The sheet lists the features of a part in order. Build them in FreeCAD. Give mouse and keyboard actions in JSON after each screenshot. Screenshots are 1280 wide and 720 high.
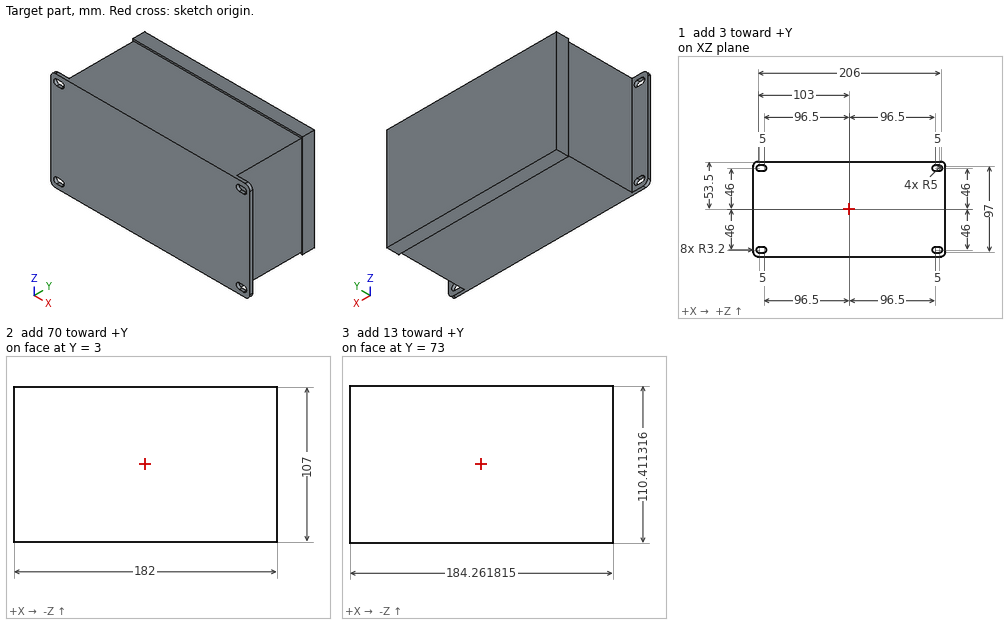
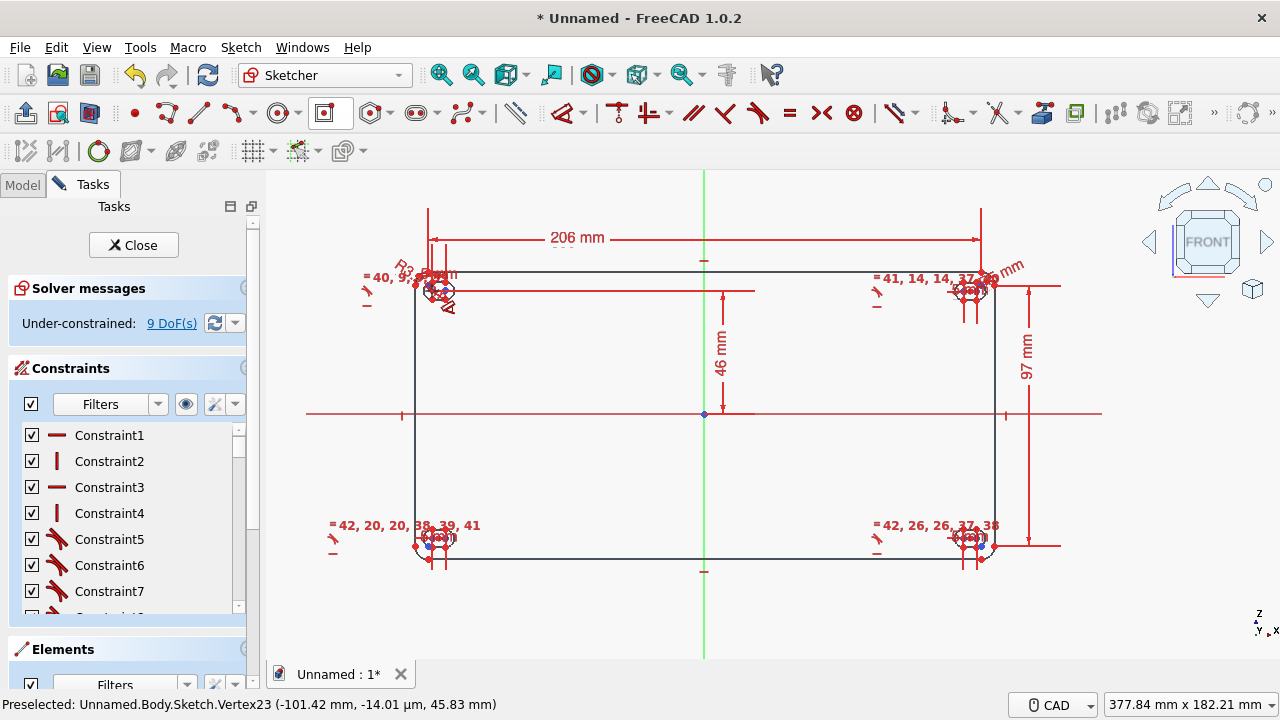
{"action": "scroll", "coordinate": [964, 292], "scroll_direction": "up", "scroll_amount": 2}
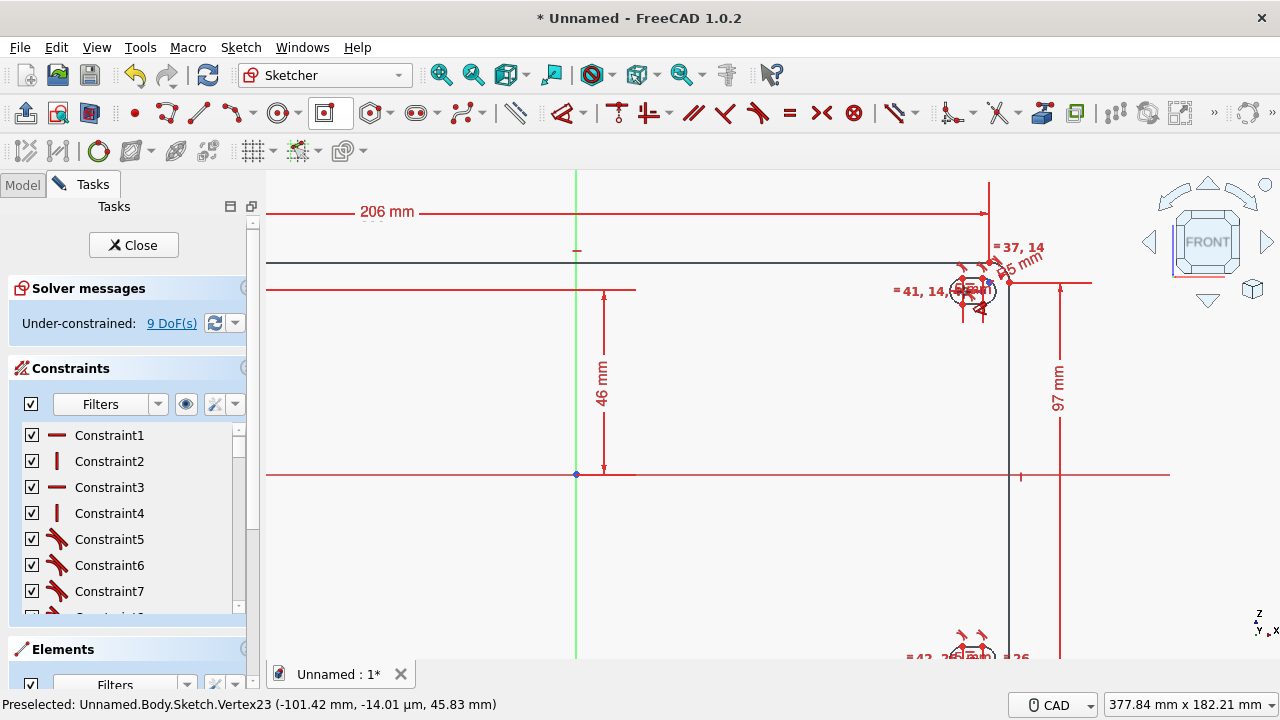
{"action": "left_click", "coordinate": [963, 291]}
{"action": "left_click", "coordinate": [542, 341]}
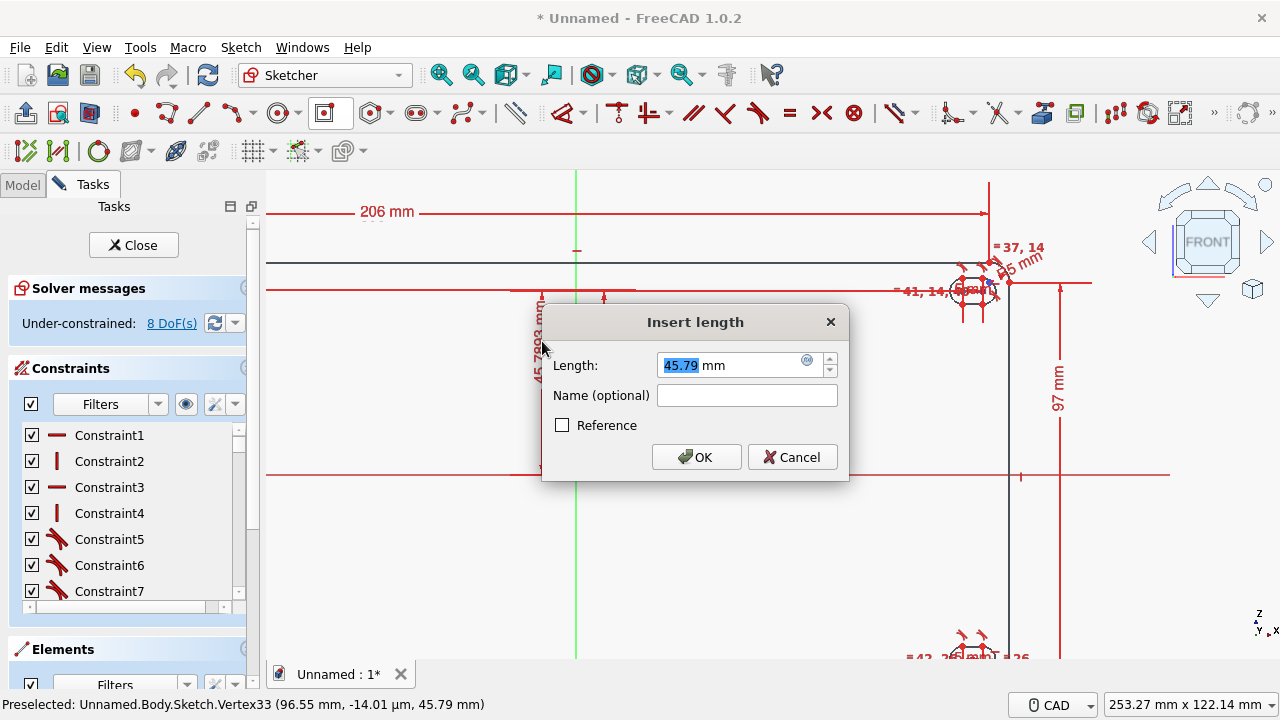
{"action": "type", "text": "46"}
{"action": "key", "text": "Return"}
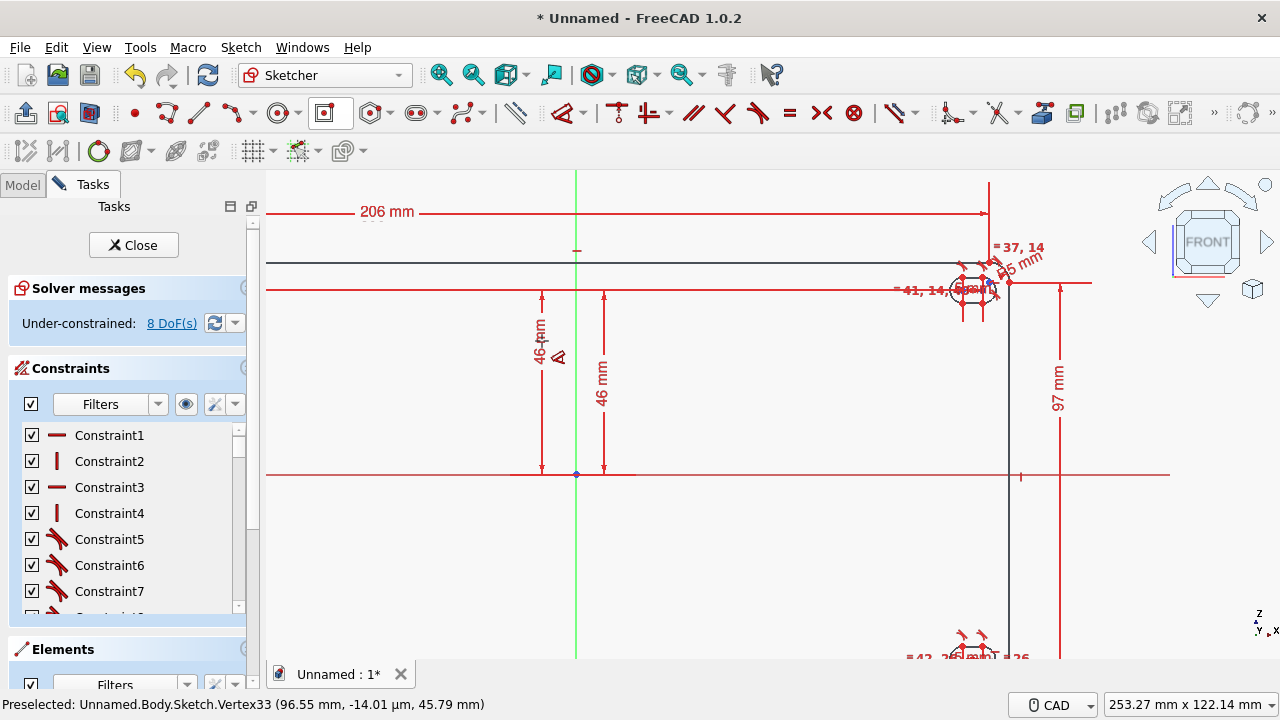
{"action": "scroll", "coordinate": [965, 292], "scroll_direction": "down", "scroll_amount": 2}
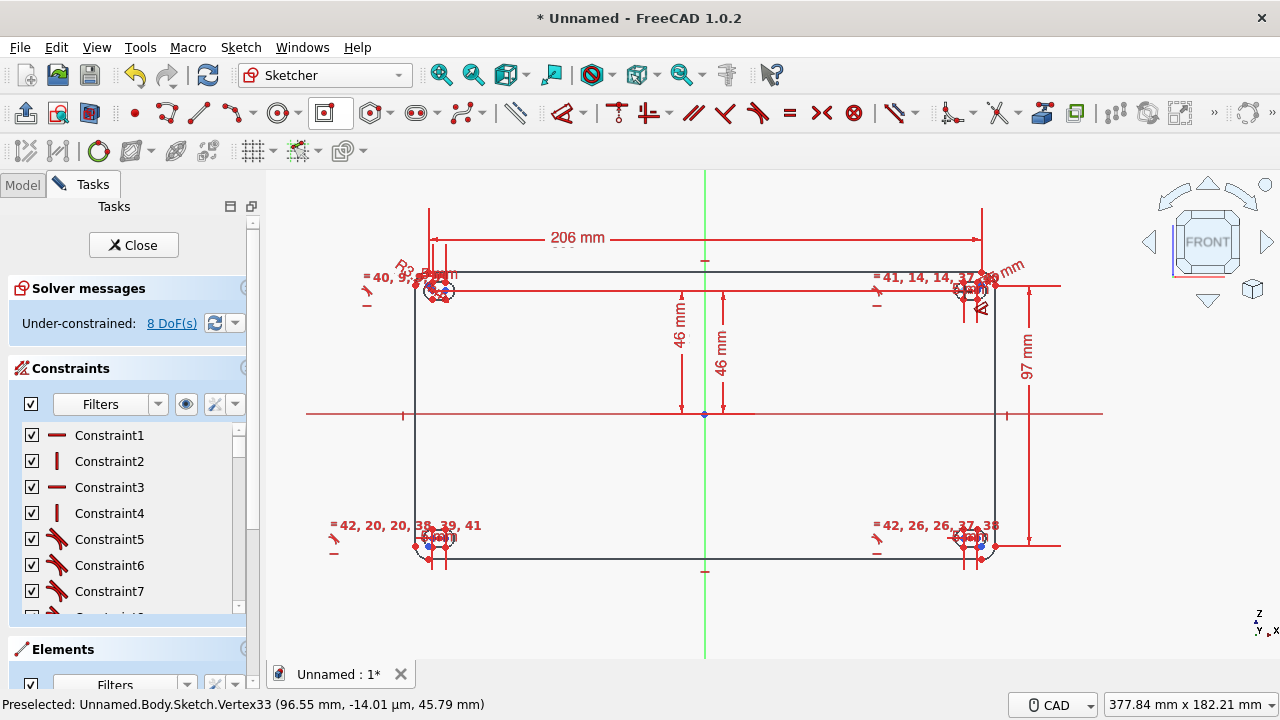
{"action": "scroll", "coordinate": [432, 539], "scroll_direction": "up", "scroll_amount": 2}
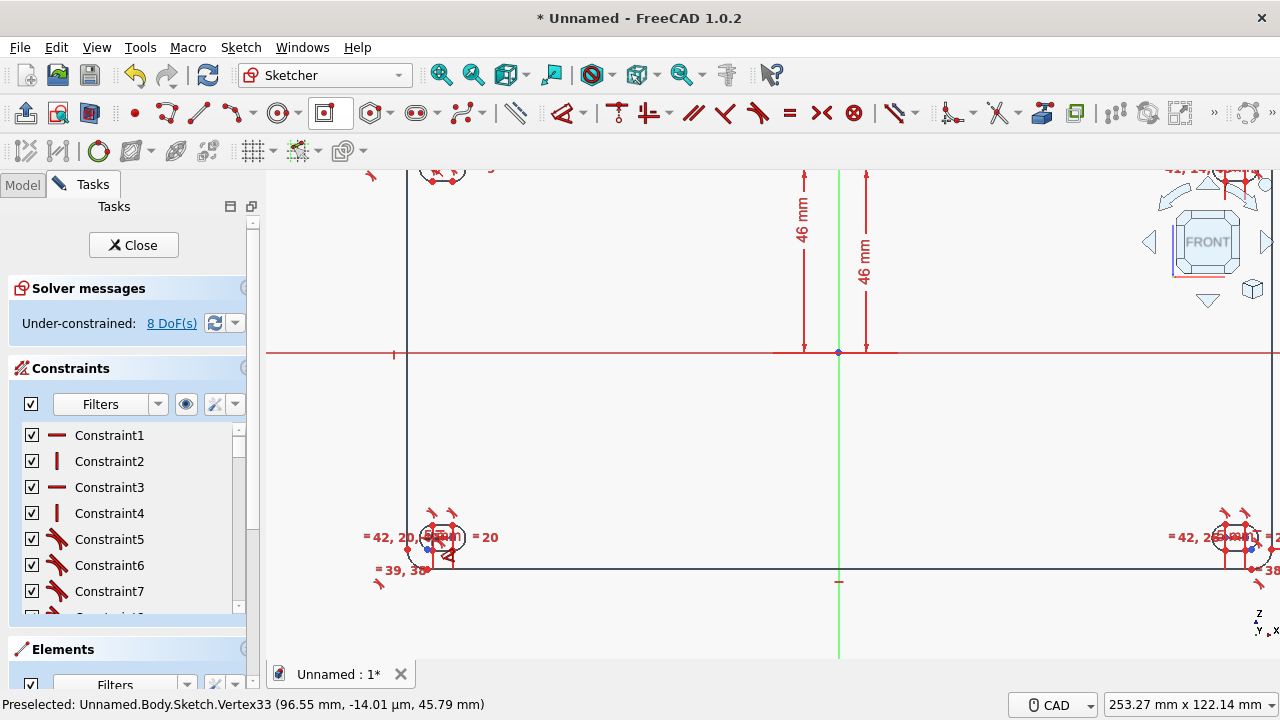
{"action": "left_click", "coordinate": [433, 538]}
{"action": "left_click", "coordinate": [873, 445]}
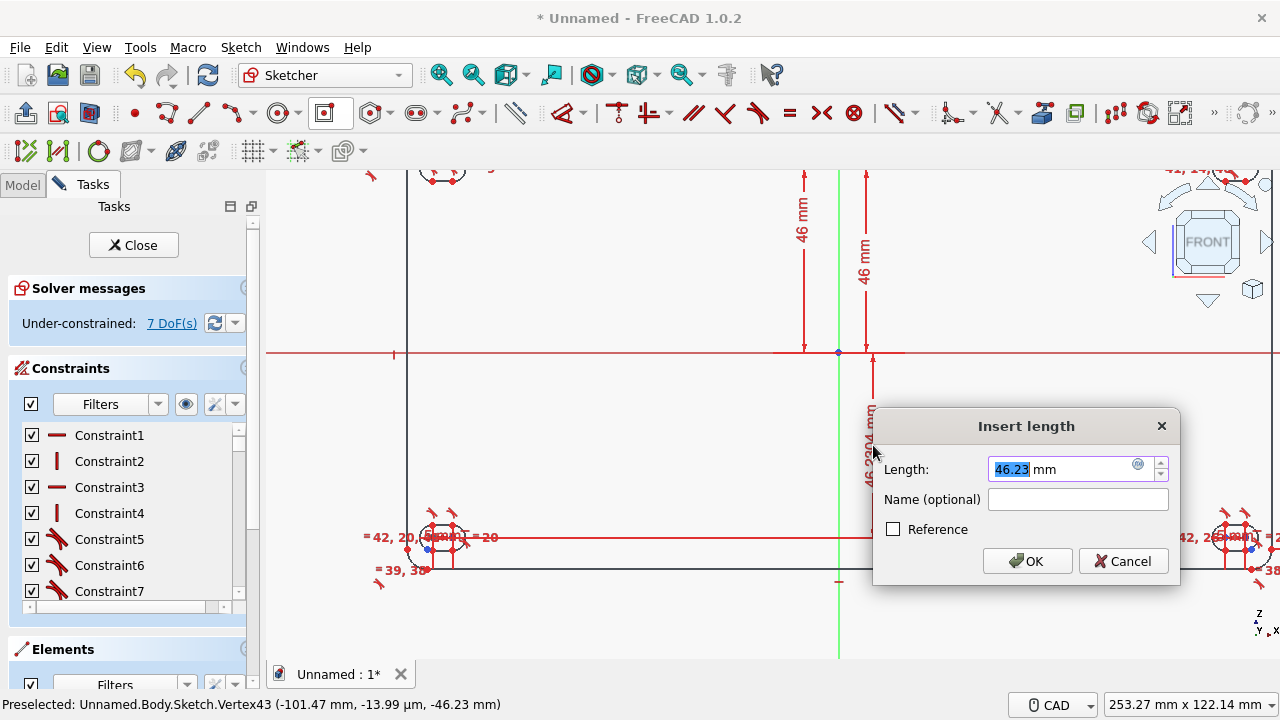
{"action": "type", "text": "46"}
{"action": "key", "text": "Return"}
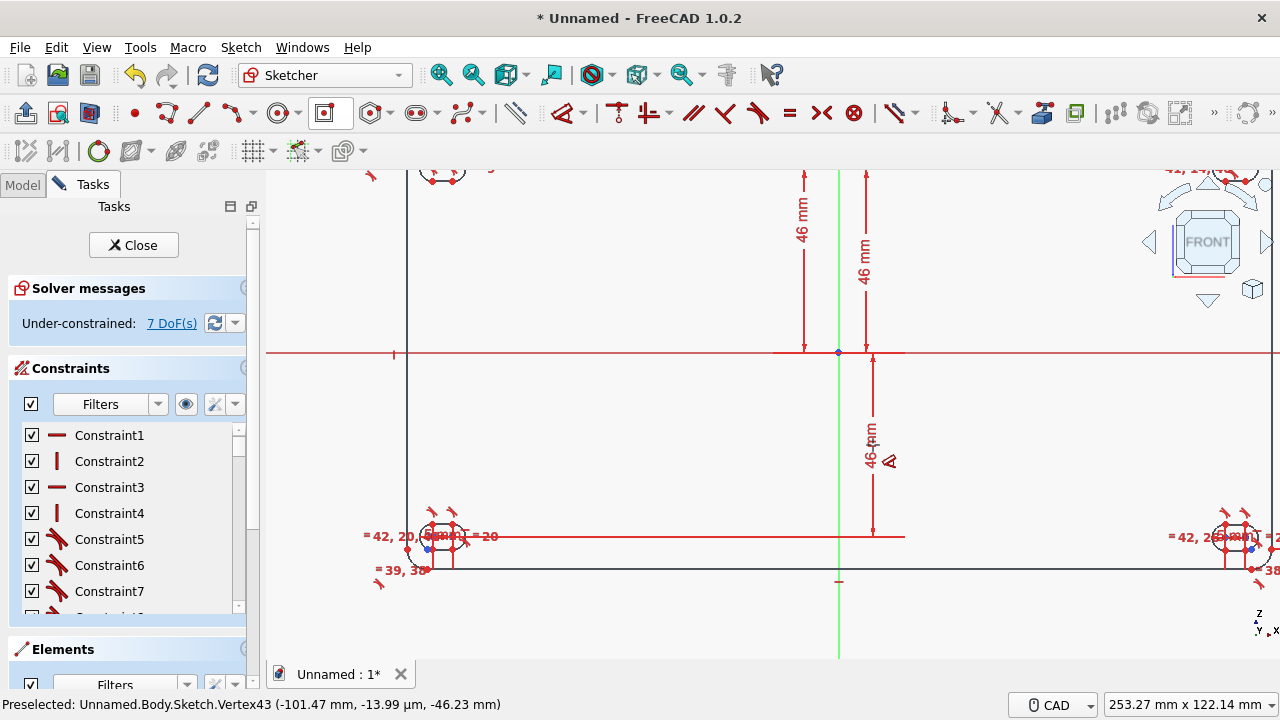
{"action": "scroll", "coordinate": [431, 540], "scroll_direction": "down", "scroll_amount": 2}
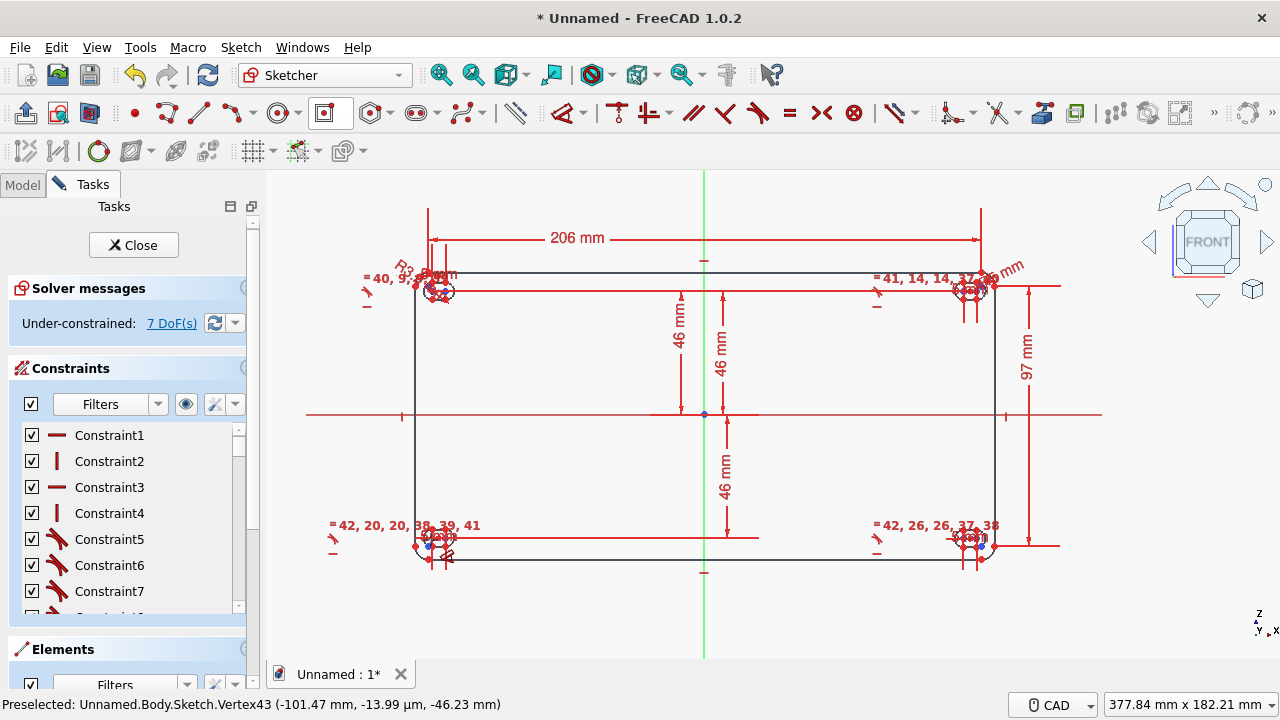
{"action": "scroll", "coordinate": [963, 539], "scroll_direction": "up", "scroll_amount": 2}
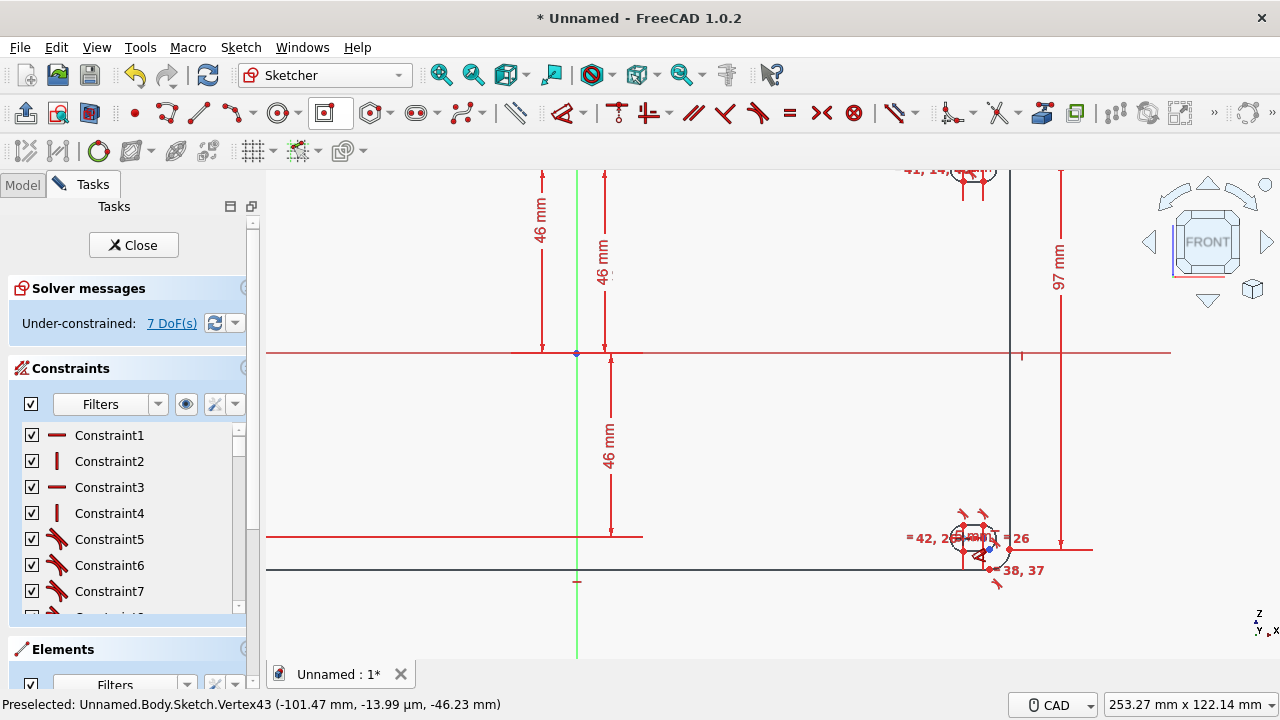
{"action": "left_click", "coordinate": [963, 538]}
{"action": "left_click", "coordinate": [543, 403]}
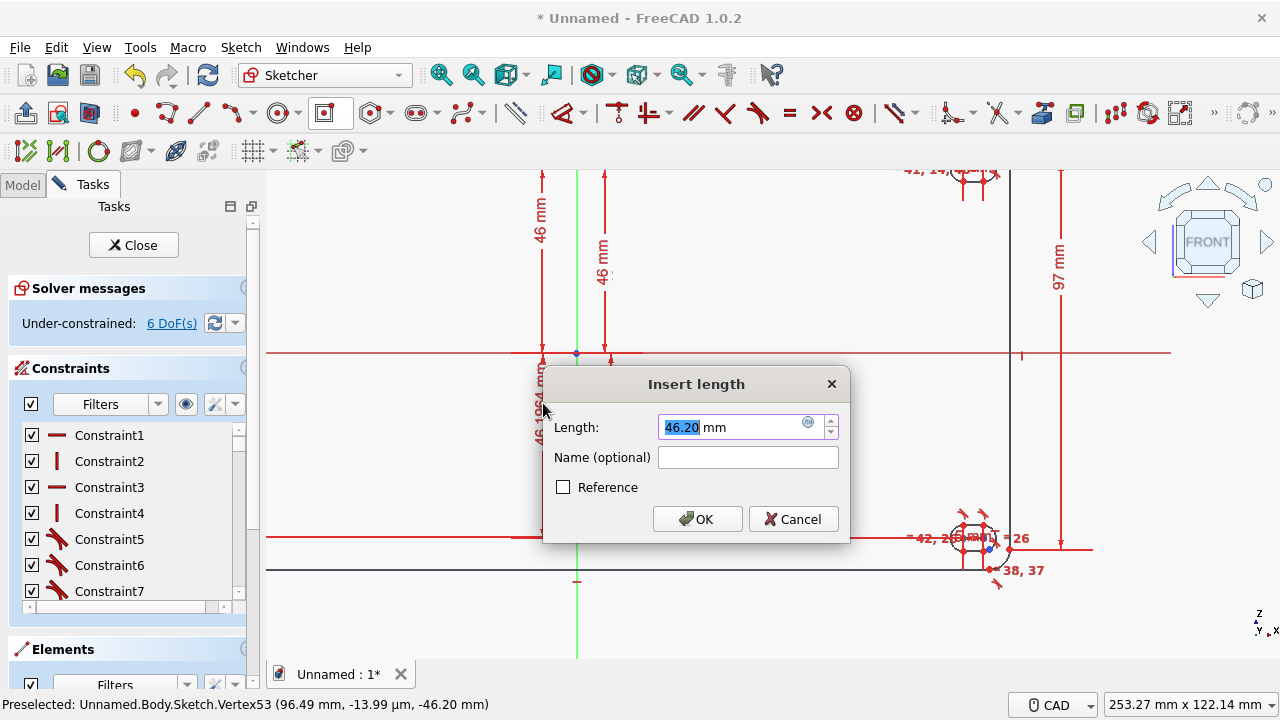
{"action": "type", "text": "46"}
{"action": "key", "text": "Return"}